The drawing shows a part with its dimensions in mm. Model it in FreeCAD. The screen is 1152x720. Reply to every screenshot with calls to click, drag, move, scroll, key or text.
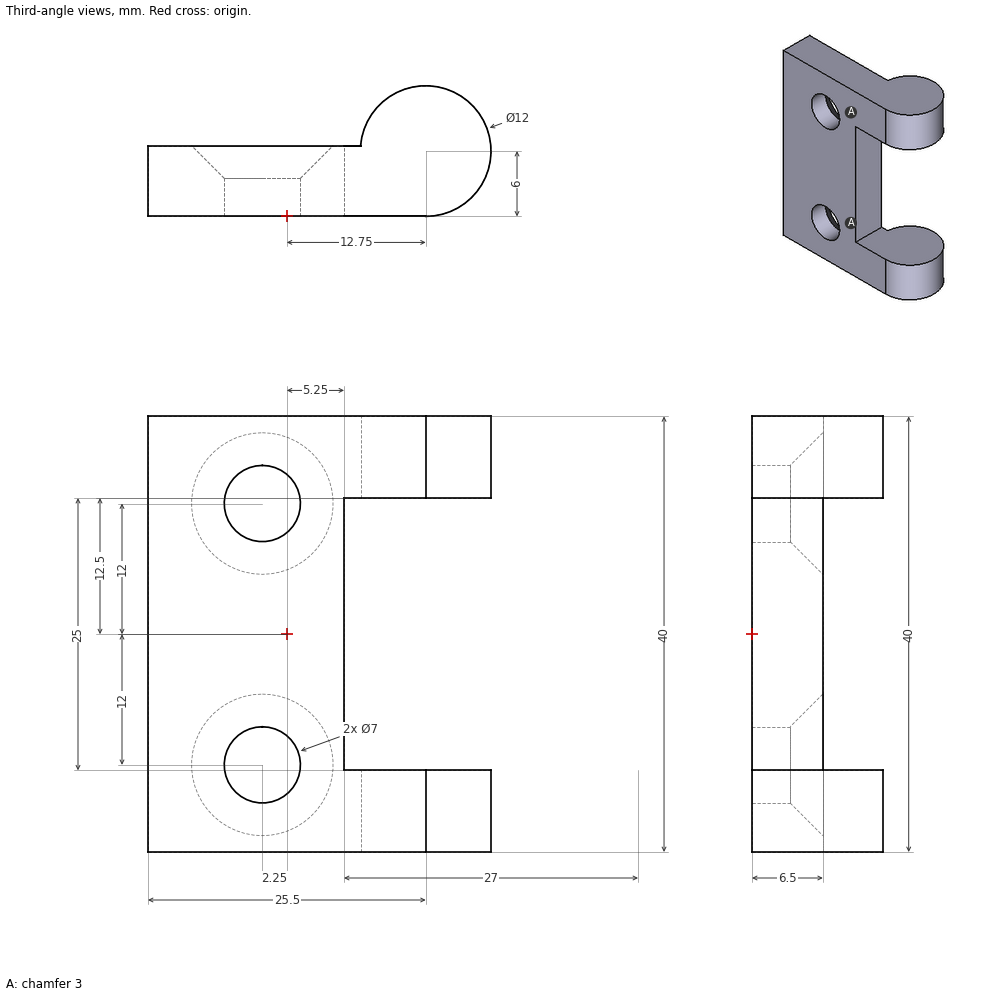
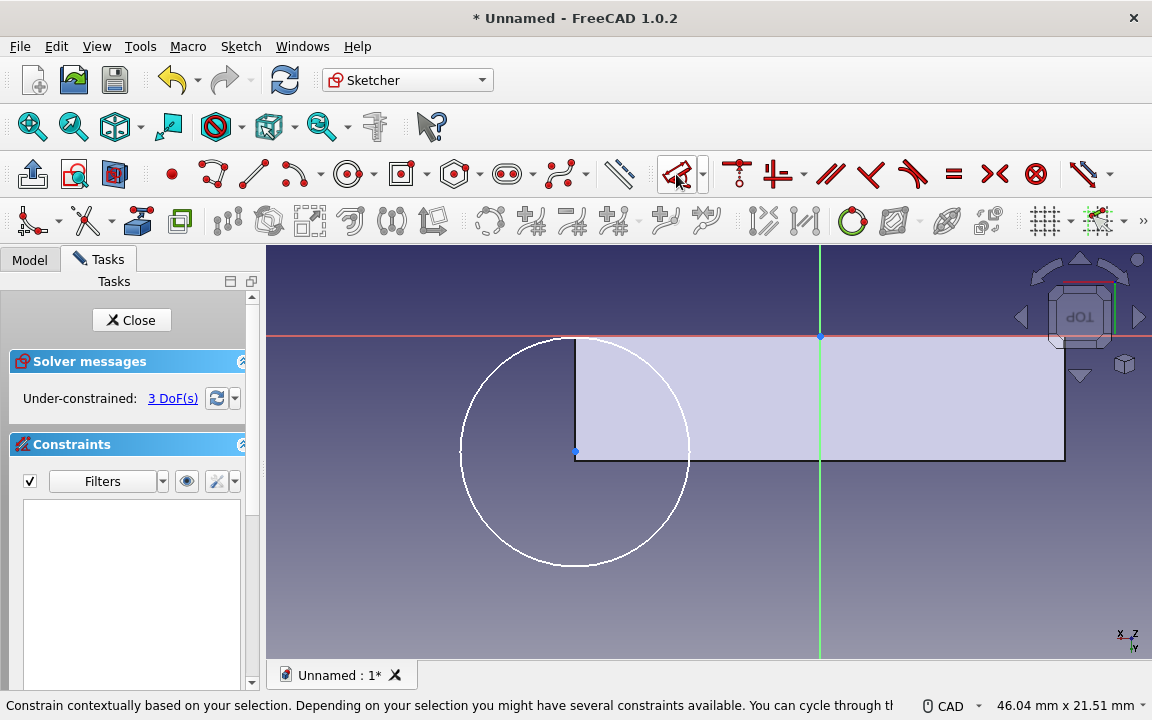
click(656, 371)
click(716, 411)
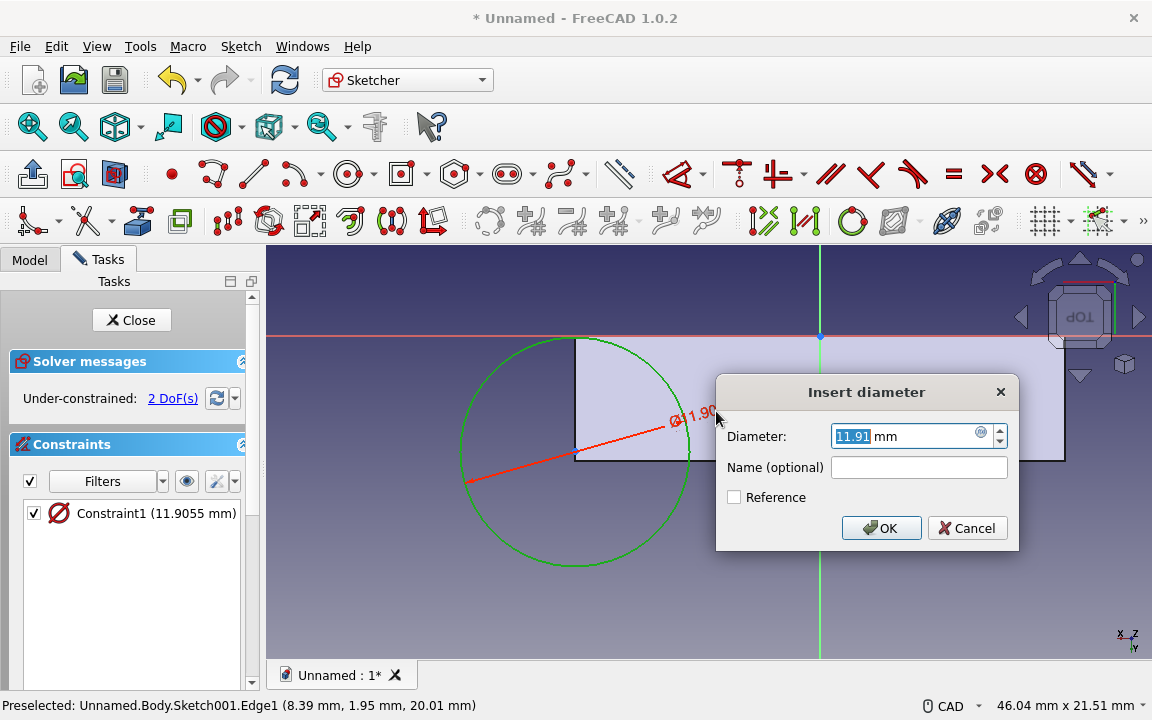
text(12)
key(Return)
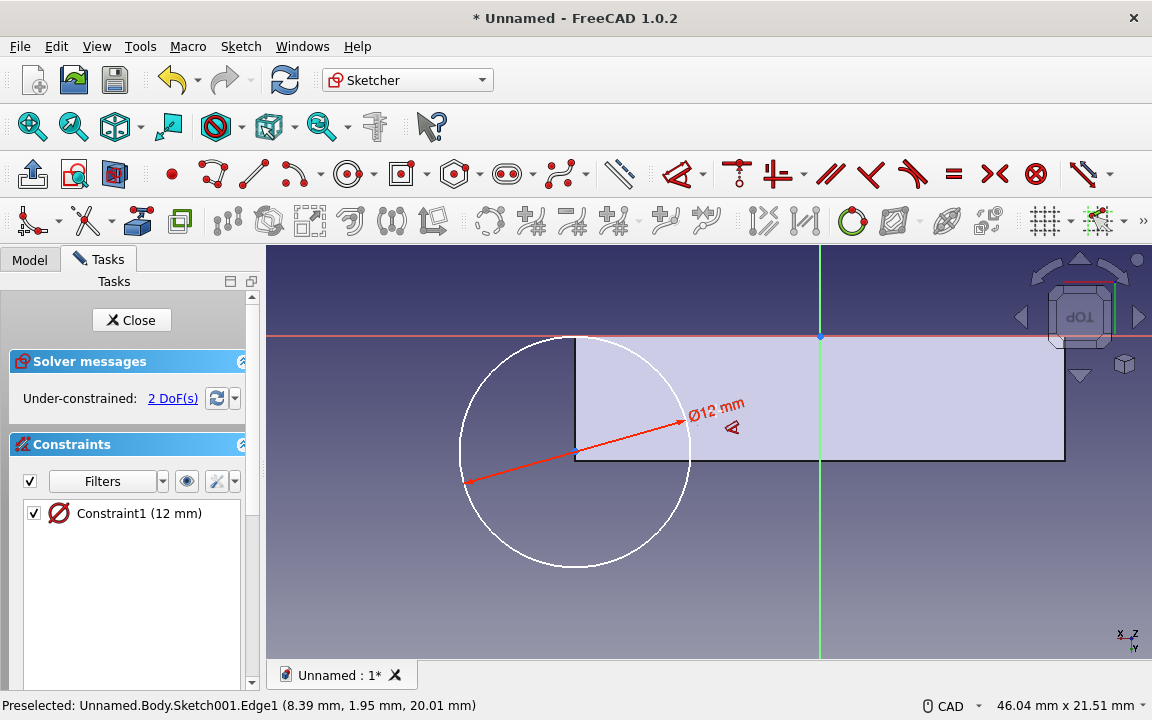
click(575, 452)
click(854, 394)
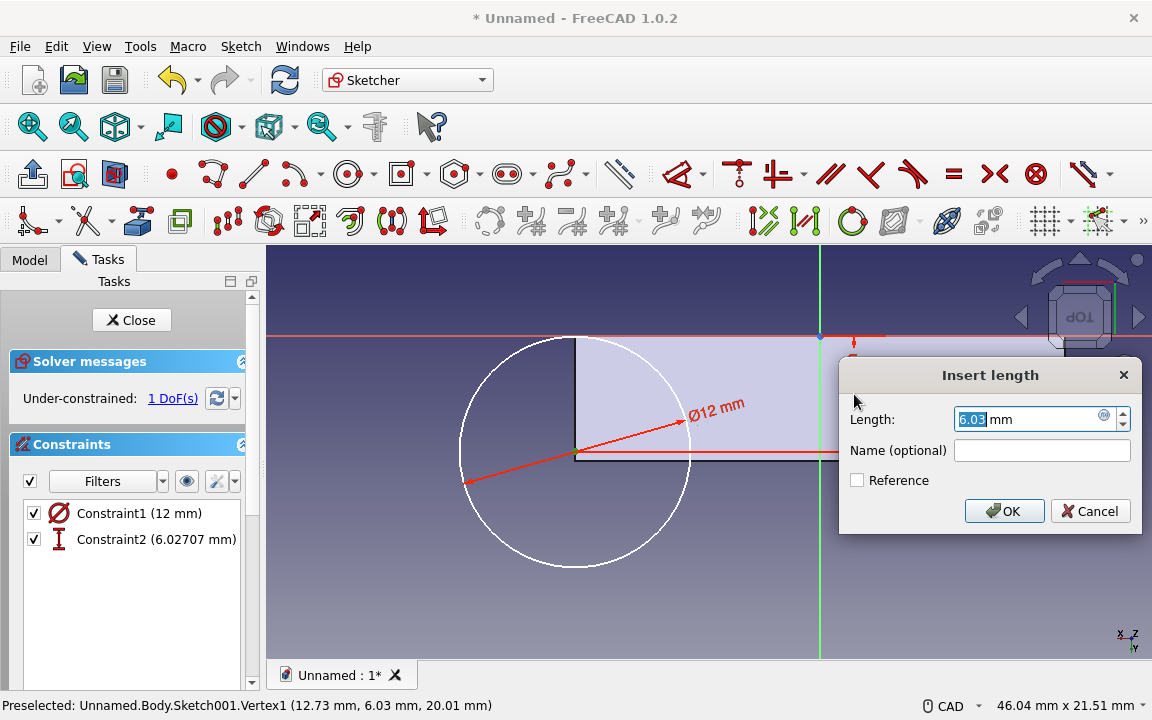
text(6)
key(Return)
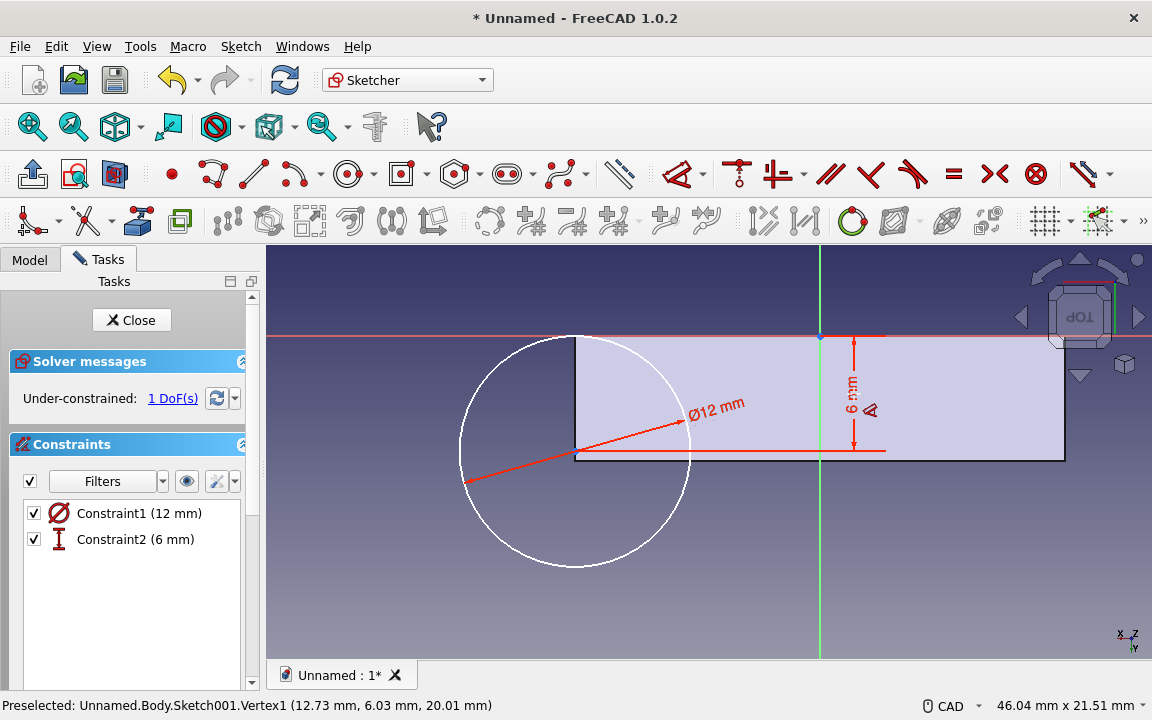
click(575, 451)
click(698, 302)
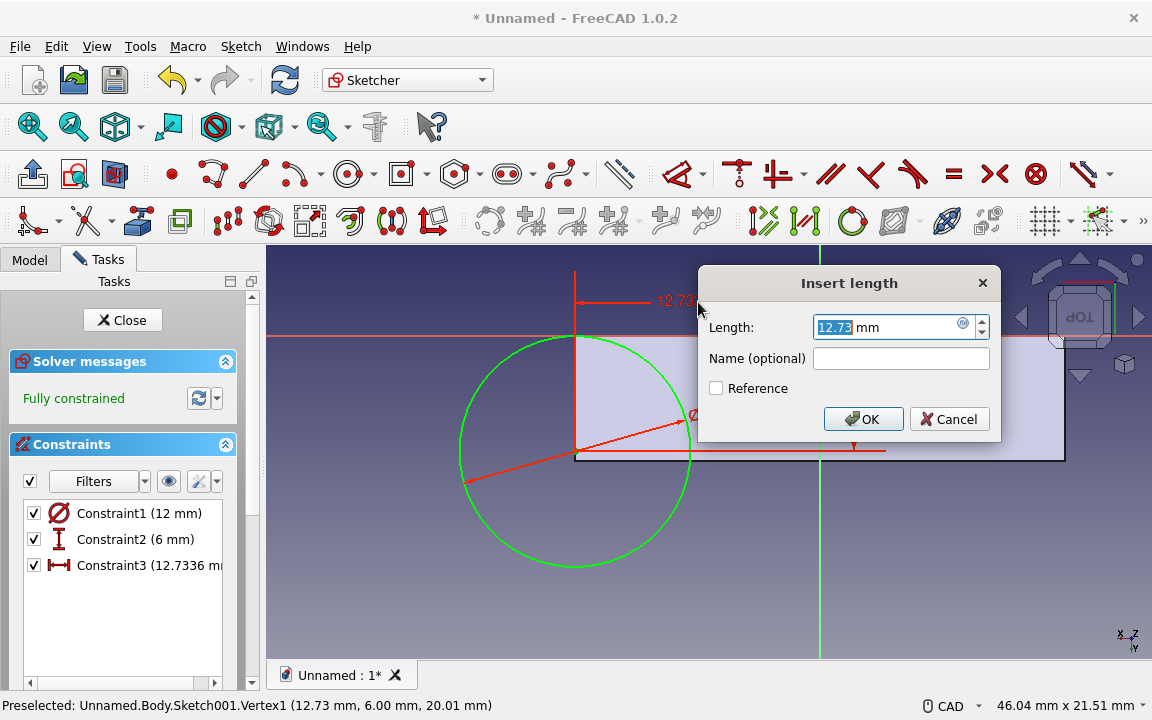
text(12.75)
key(Return)
key(Escape)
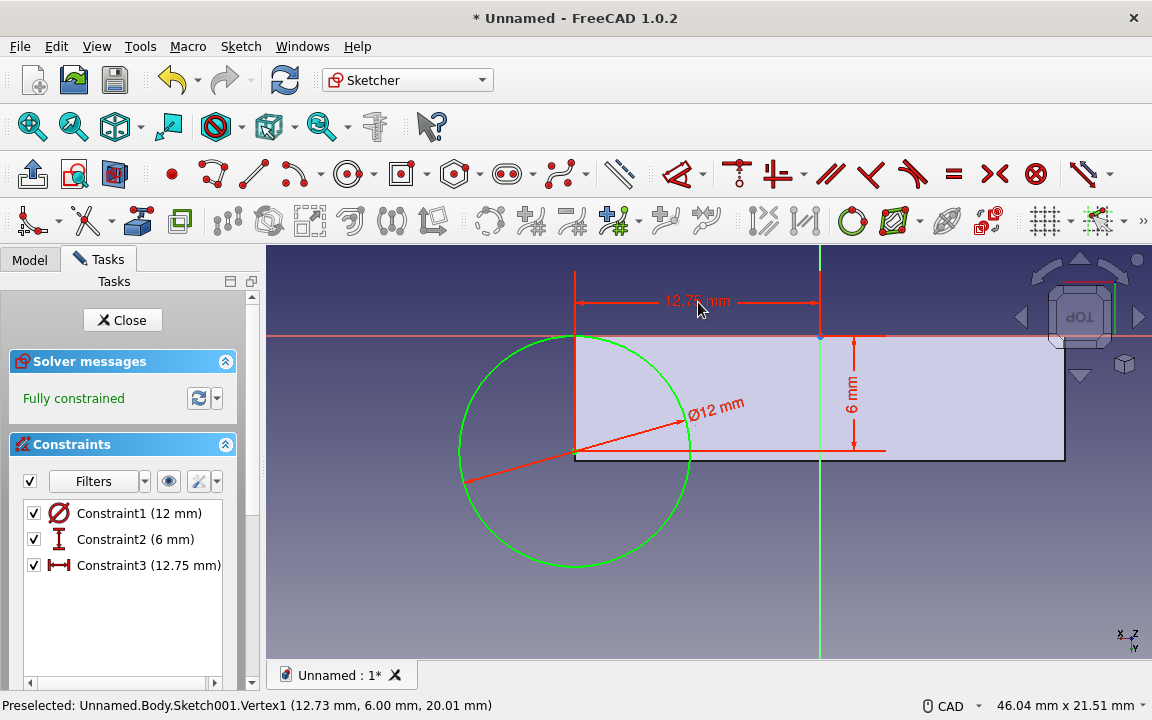
click(123, 320)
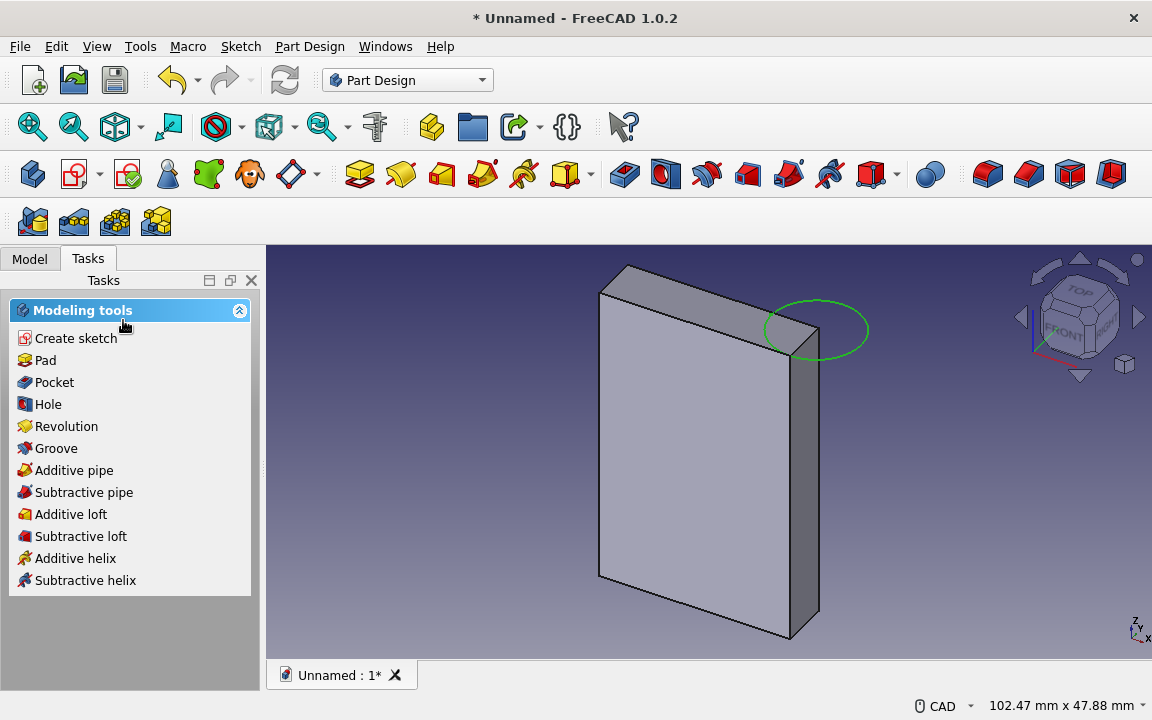
click(360, 174)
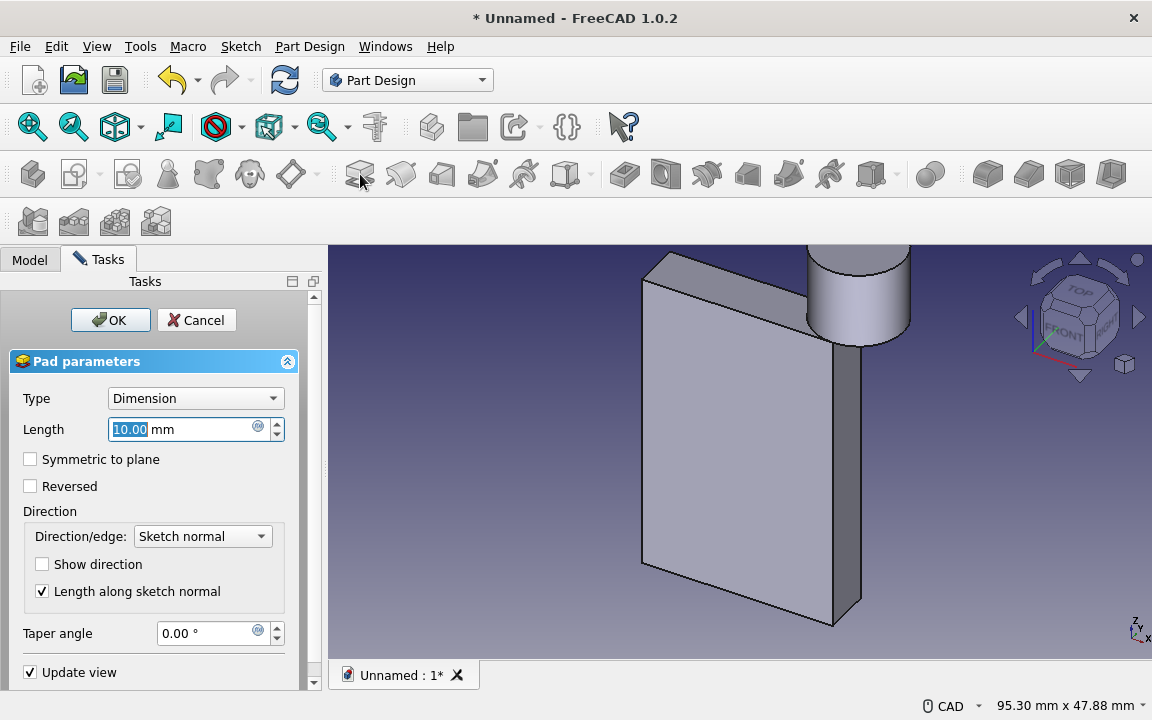
text(40)
key(Tab)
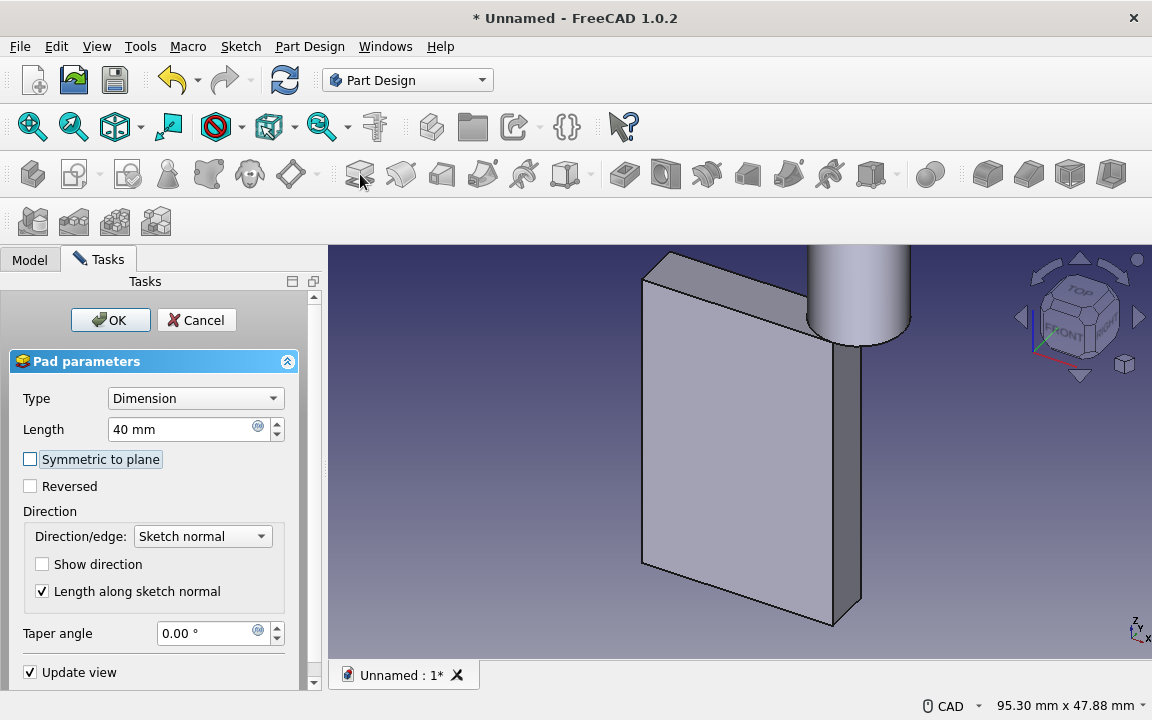
click(31, 486)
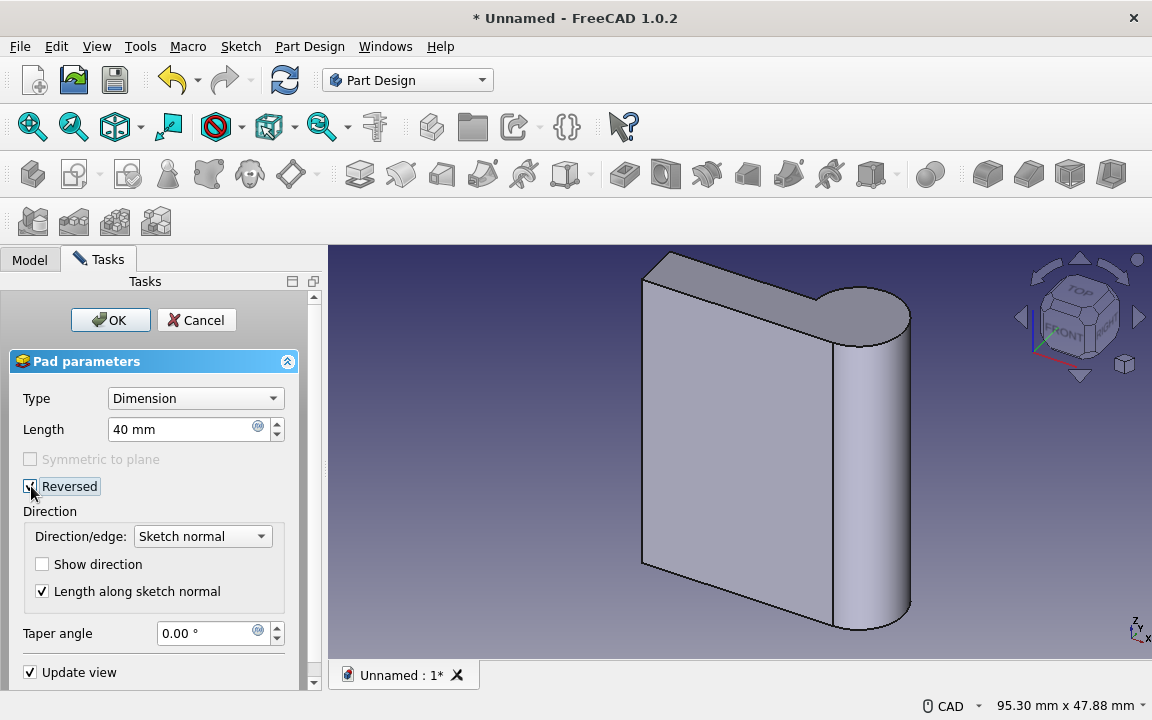
click(111, 320)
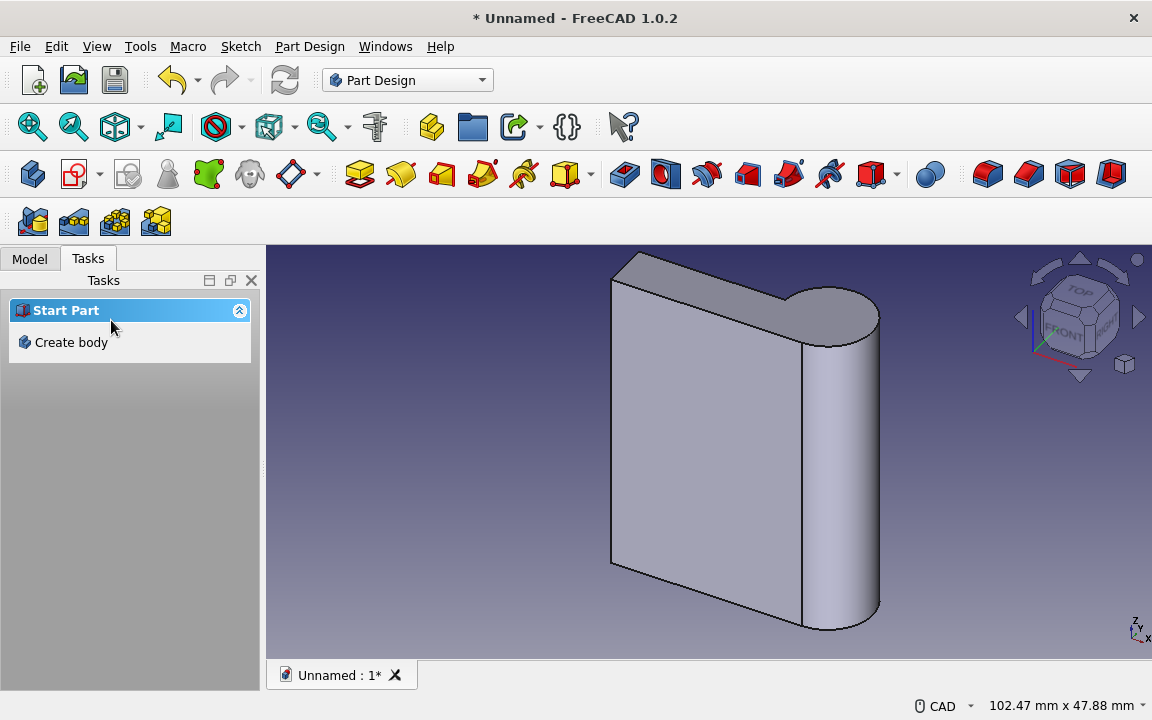
click(33, 128)